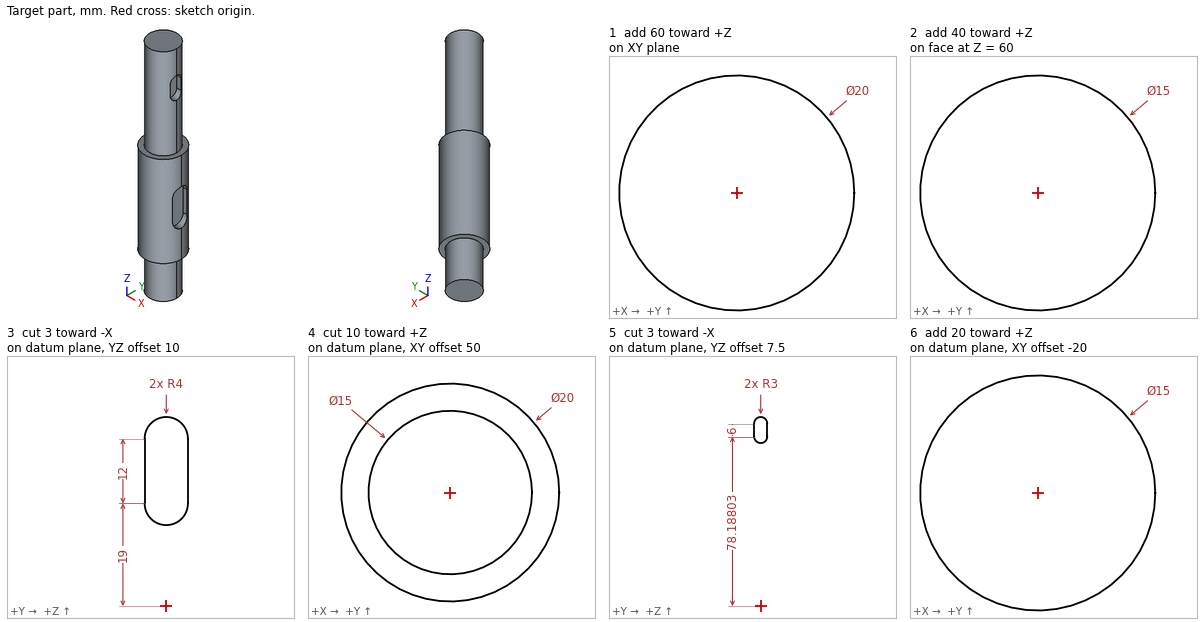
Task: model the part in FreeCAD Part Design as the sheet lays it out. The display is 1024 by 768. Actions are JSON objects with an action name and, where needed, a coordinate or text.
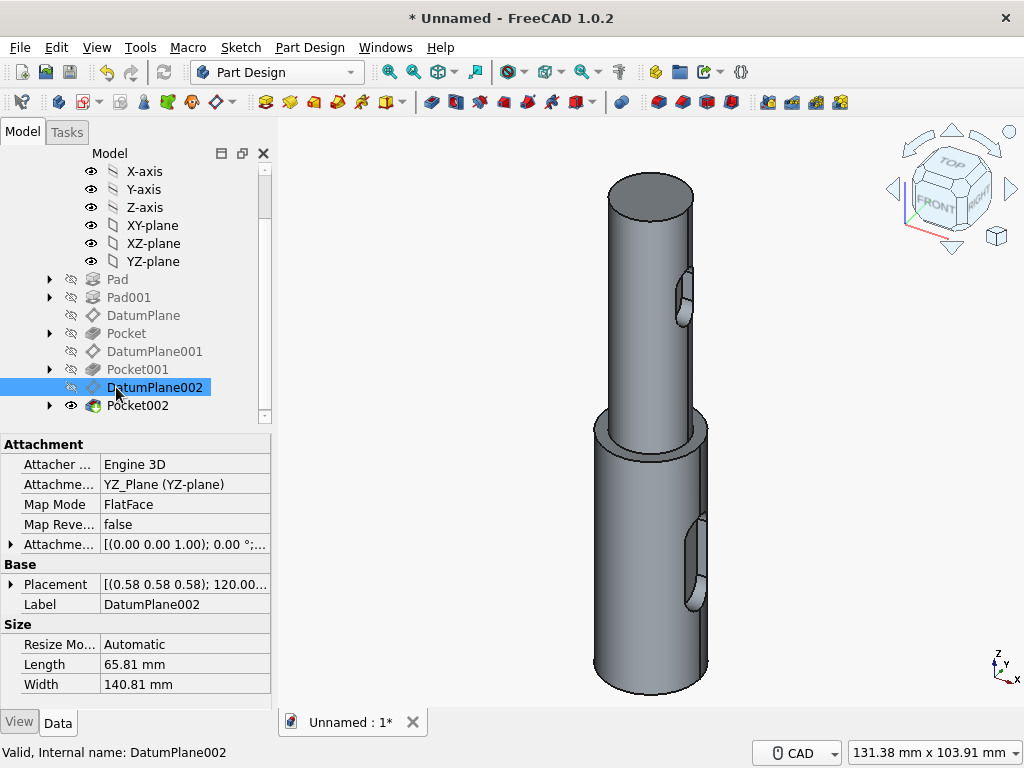
{"action": "scroll", "coordinate": [160, 293], "scroll_direction": "down", "scroll_amount": 3}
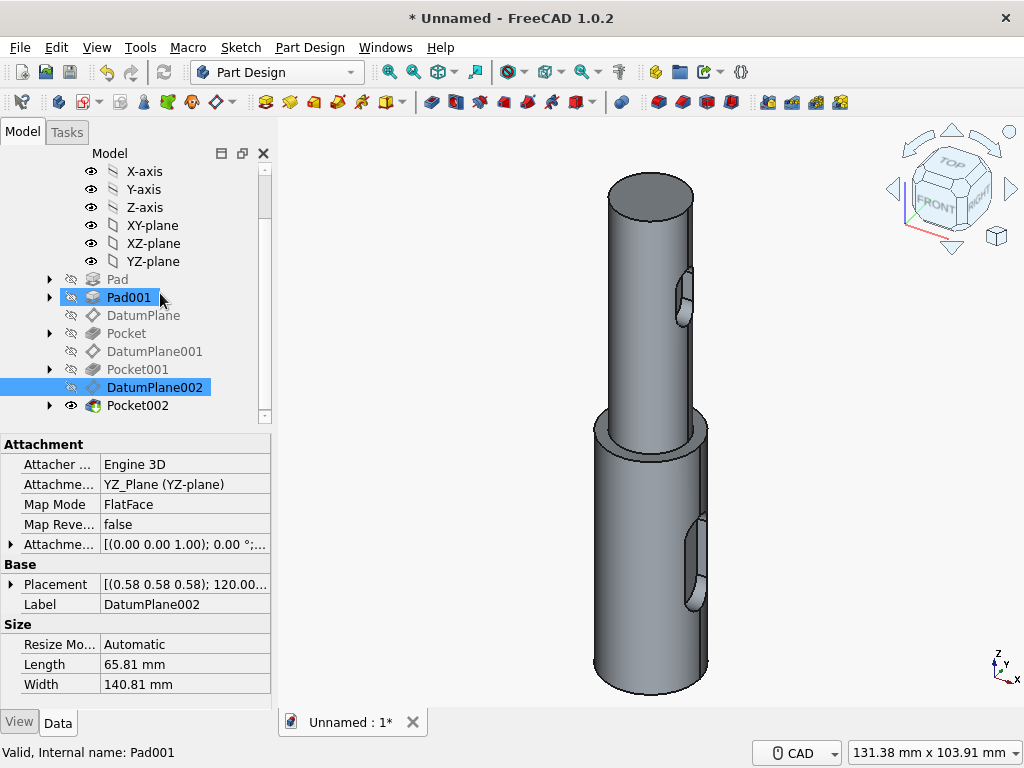
{"action": "scroll", "coordinate": [160, 293], "scroll_direction": "up", "scroll_amount": 15}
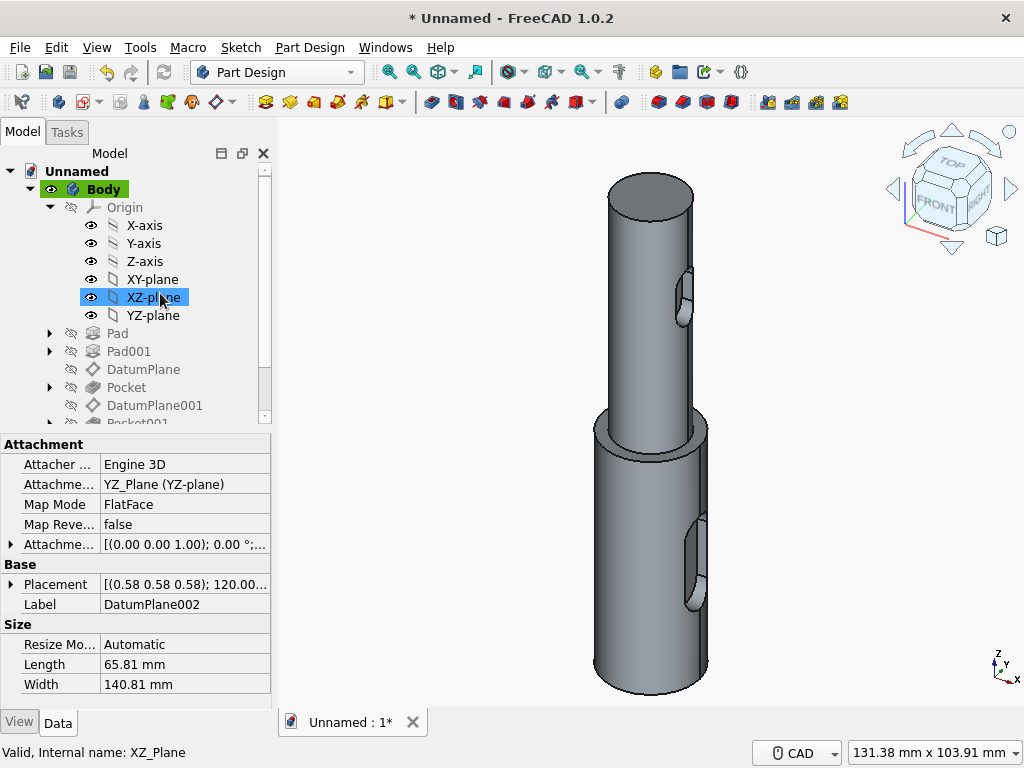
{"action": "left_click", "coordinate": [136, 279]}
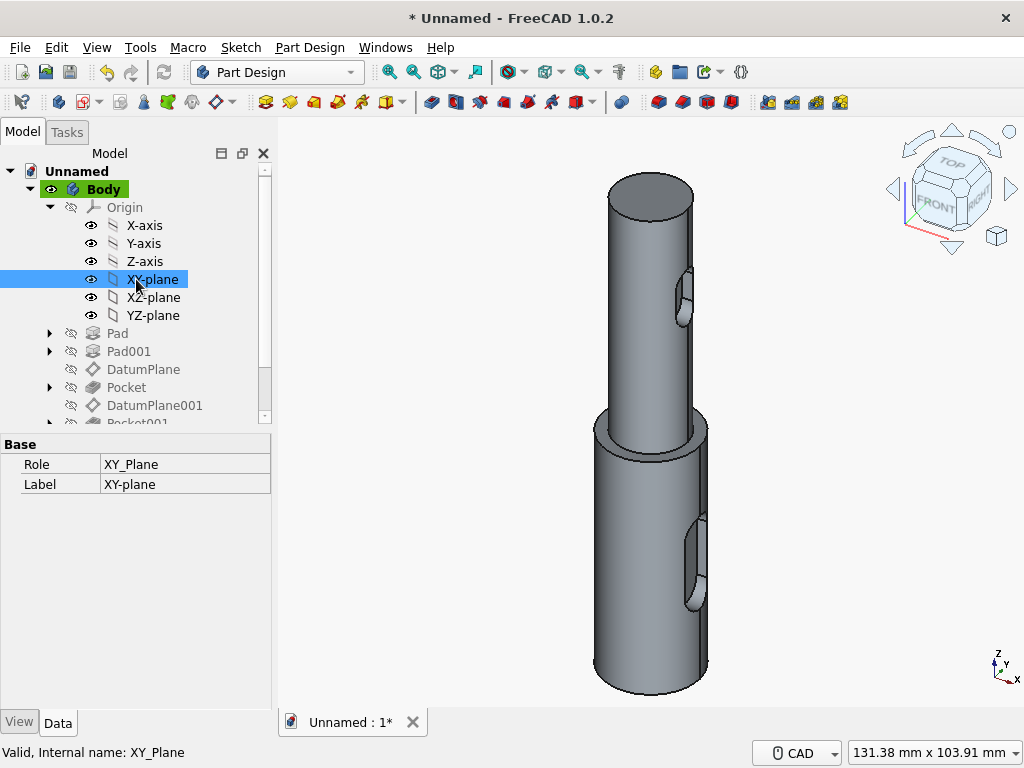
{"action": "left_click", "coordinate": [216, 102]}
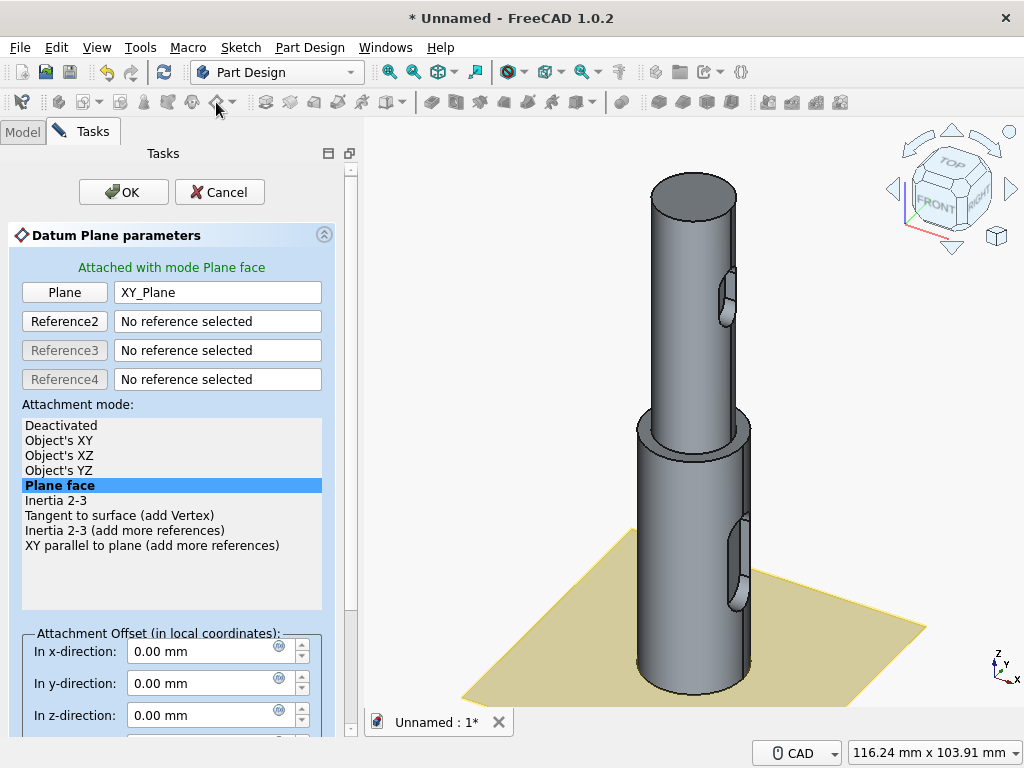
{"action": "triple_click", "coordinate": [210, 715]}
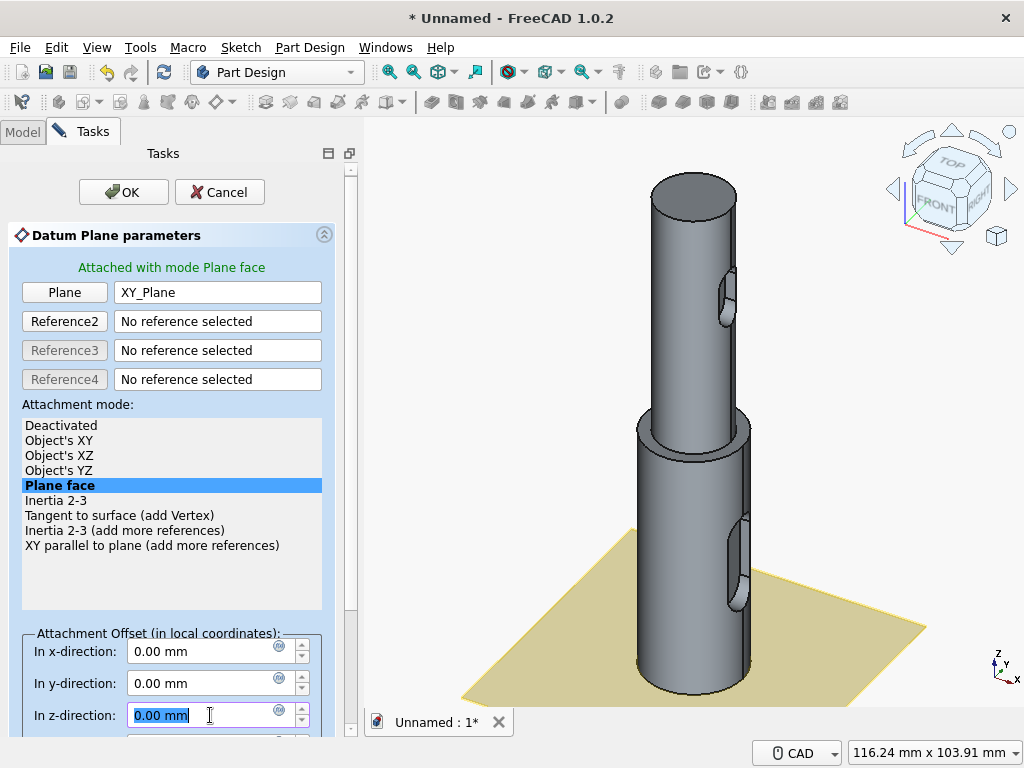
{"action": "type", "text": "-20"}
{"action": "key", "text": "Tab"}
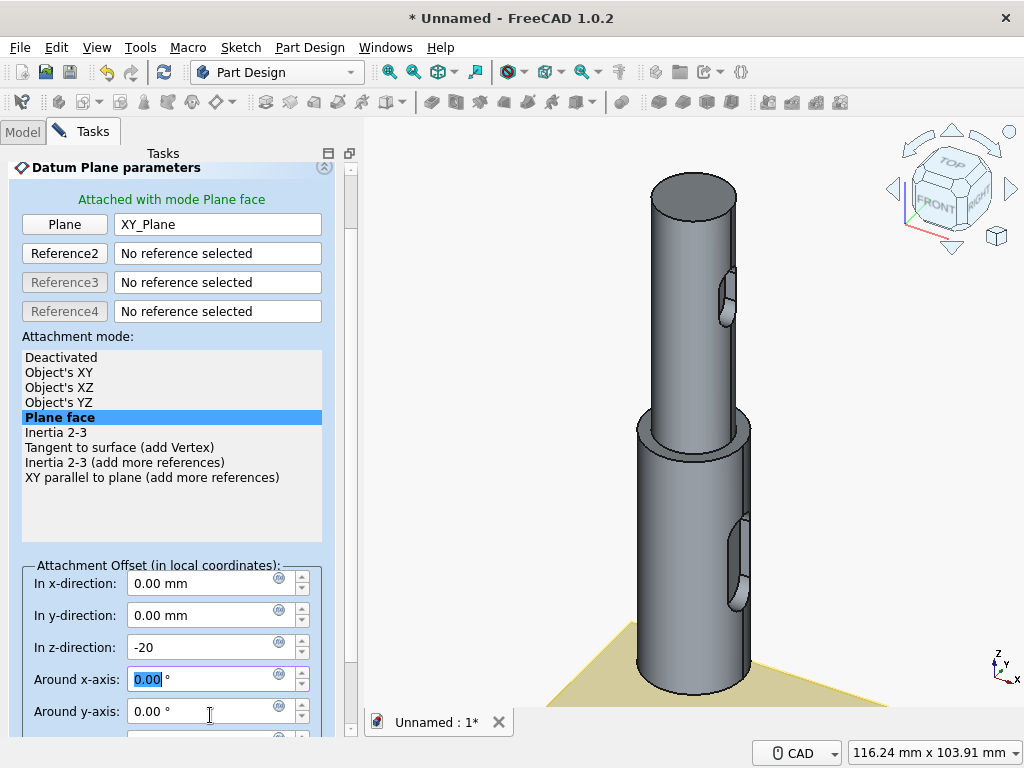
{"action": "scroll", "coordinate": [351, 450], "scroll_direction": "up", "scroll_amount": 2}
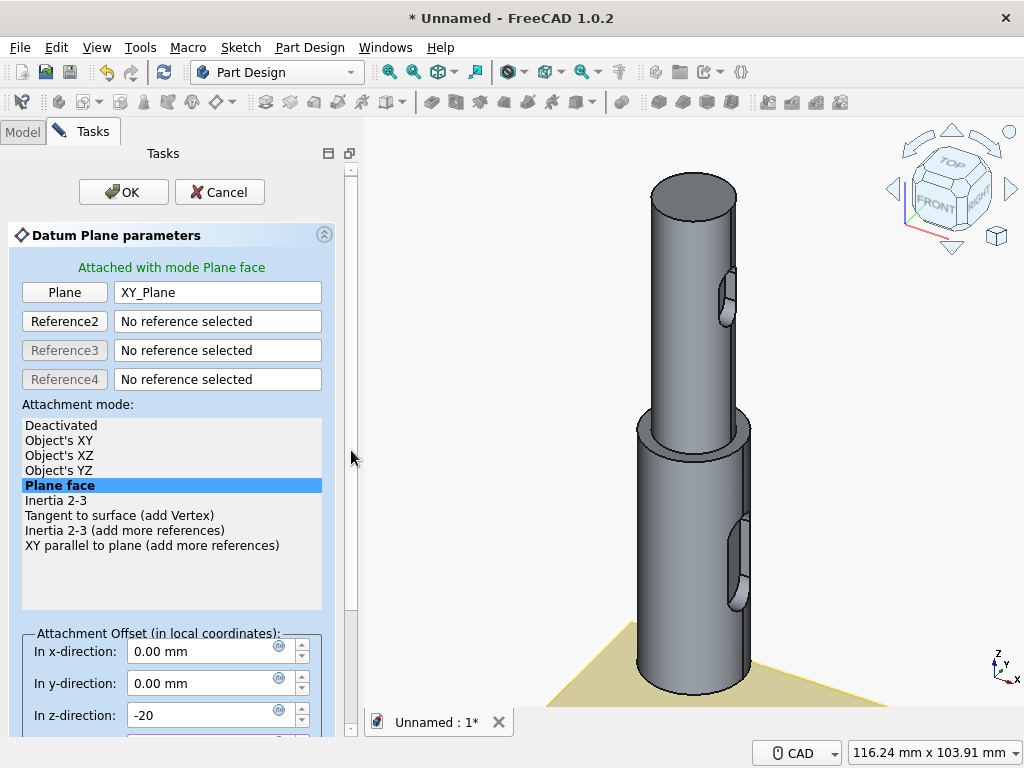
{"action": "left_click", "coordinate": [124, 192]}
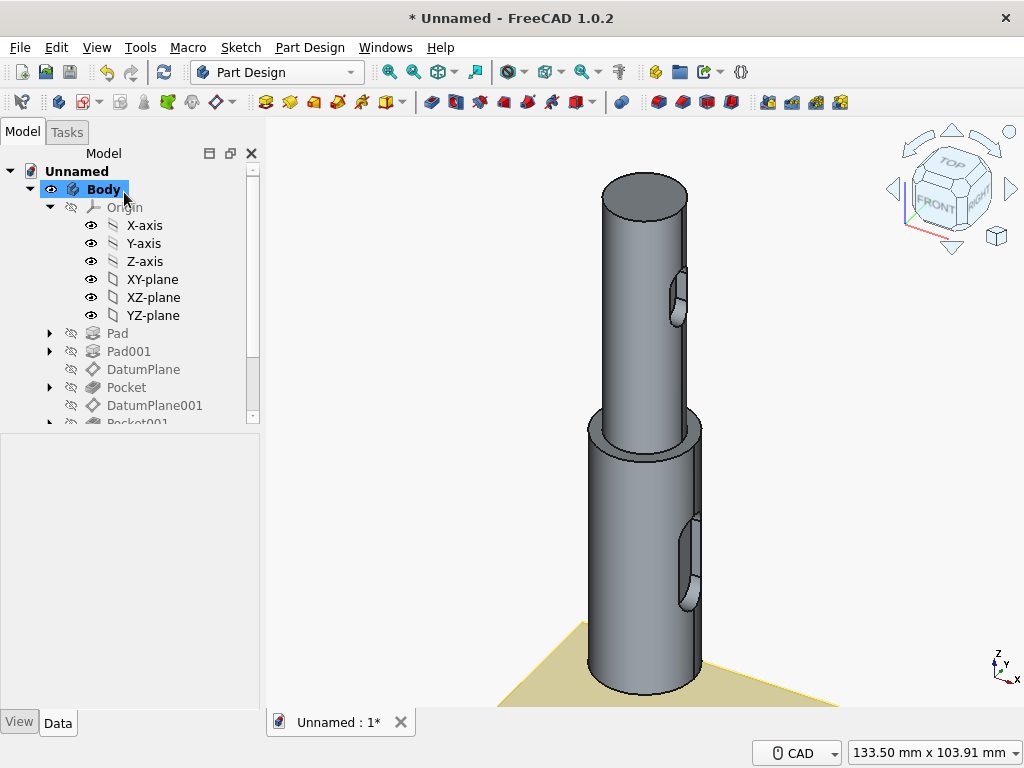
{"action": "scroll", "coordinate": [100, 293], "scroll_direction": "down", "scroll_amount": 3}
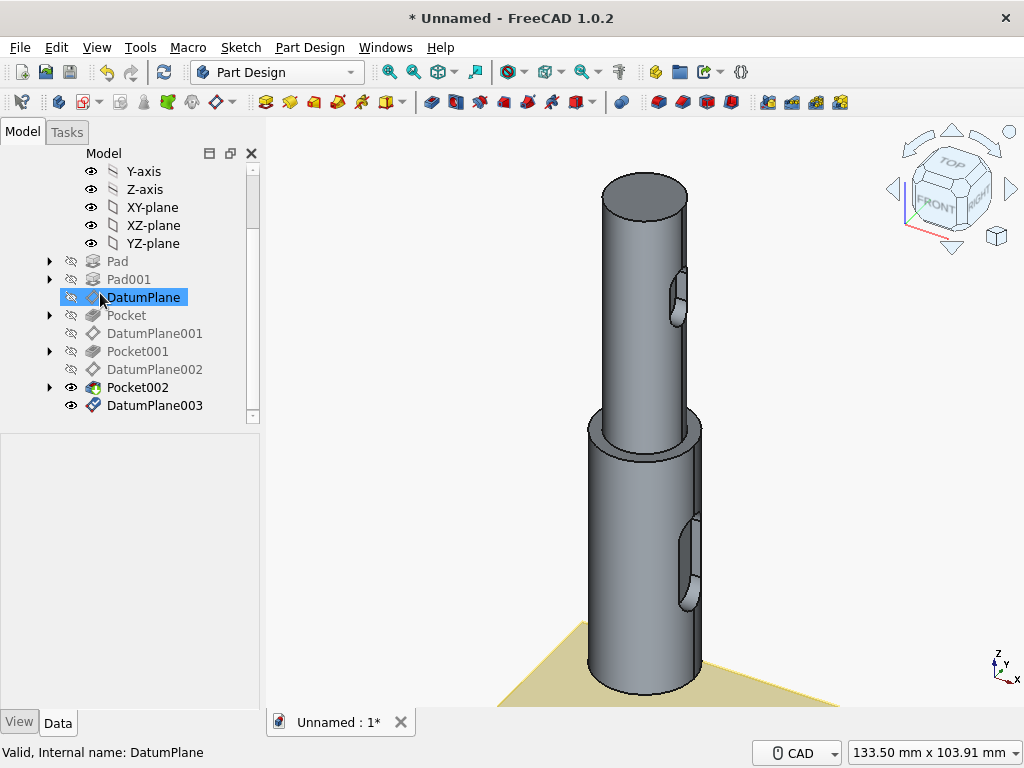
{"action": "left_click", "coordinate": [116, 405]}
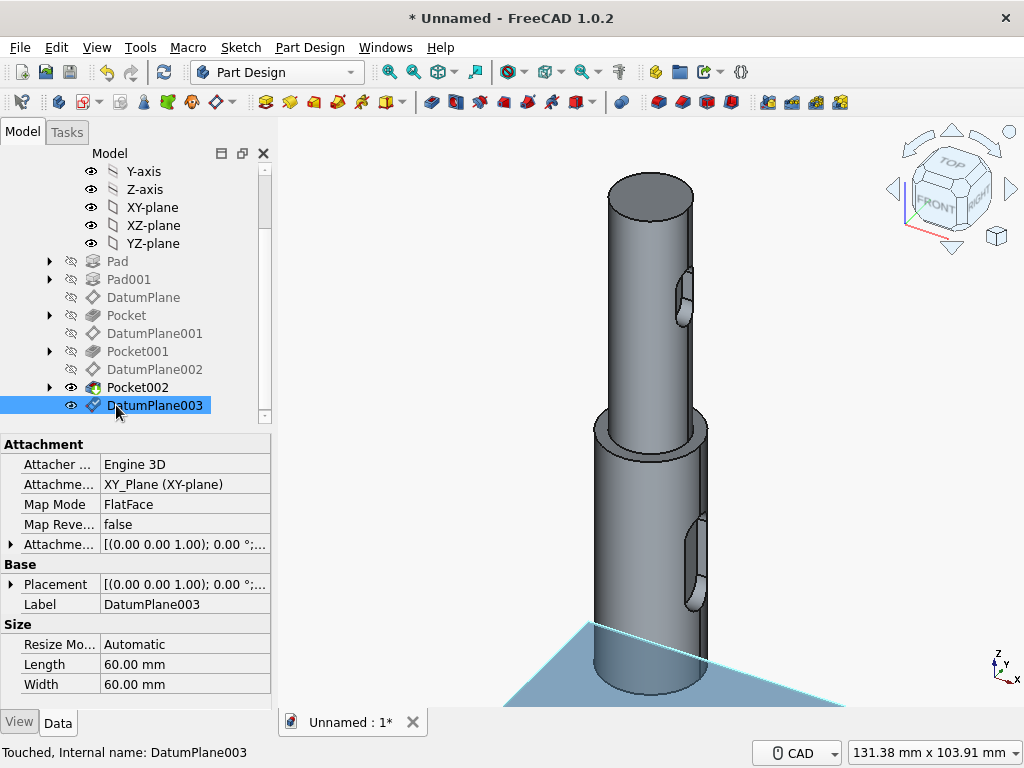
{"action": "left_click", "coordinate": [84, 102]}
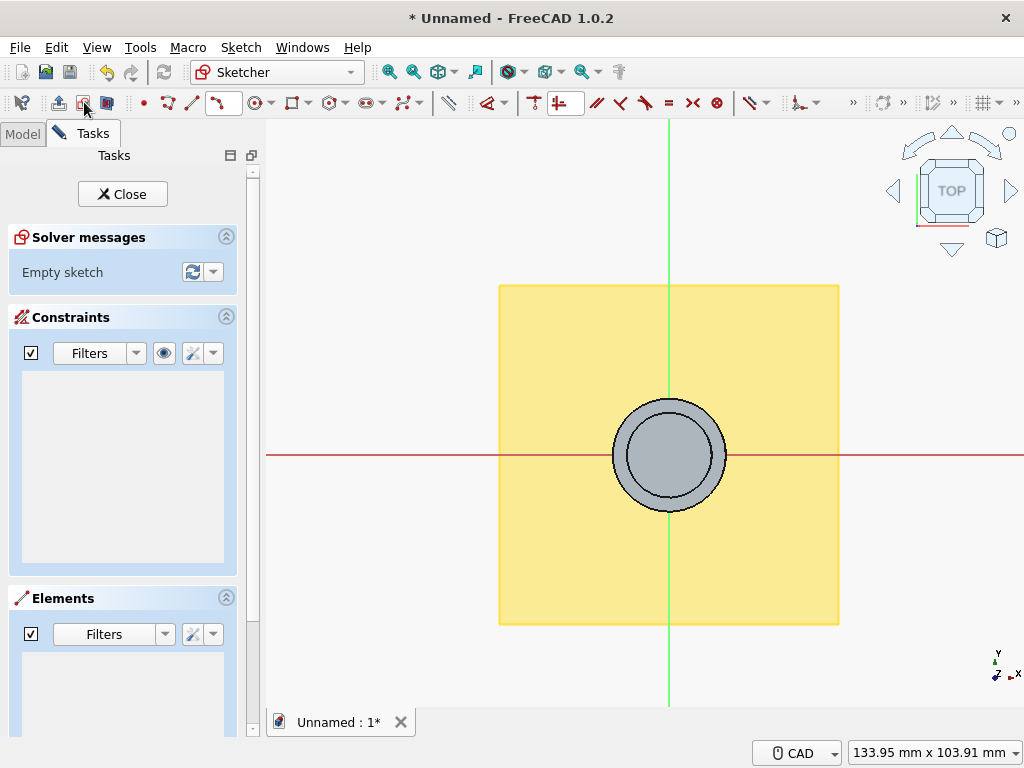
{"action": "left_click", "coordinate": [108, 104]}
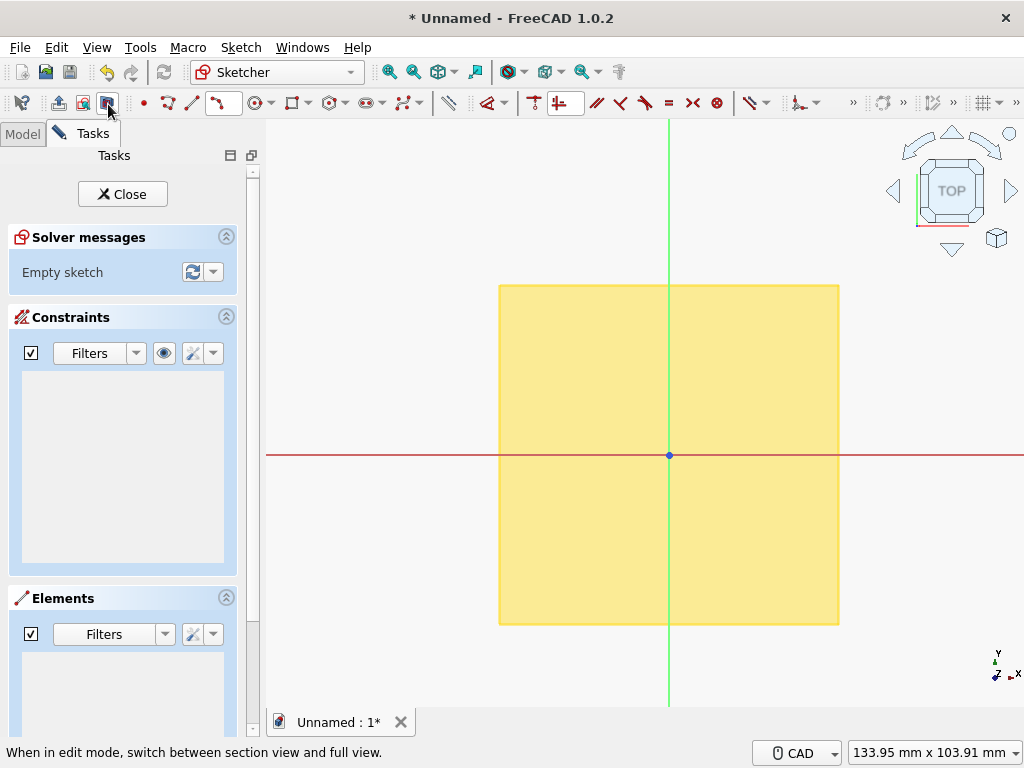
{"action": "scroll", "coordinate": [700, 469], "scroll_direction": "up", "scroll_amount": 7}